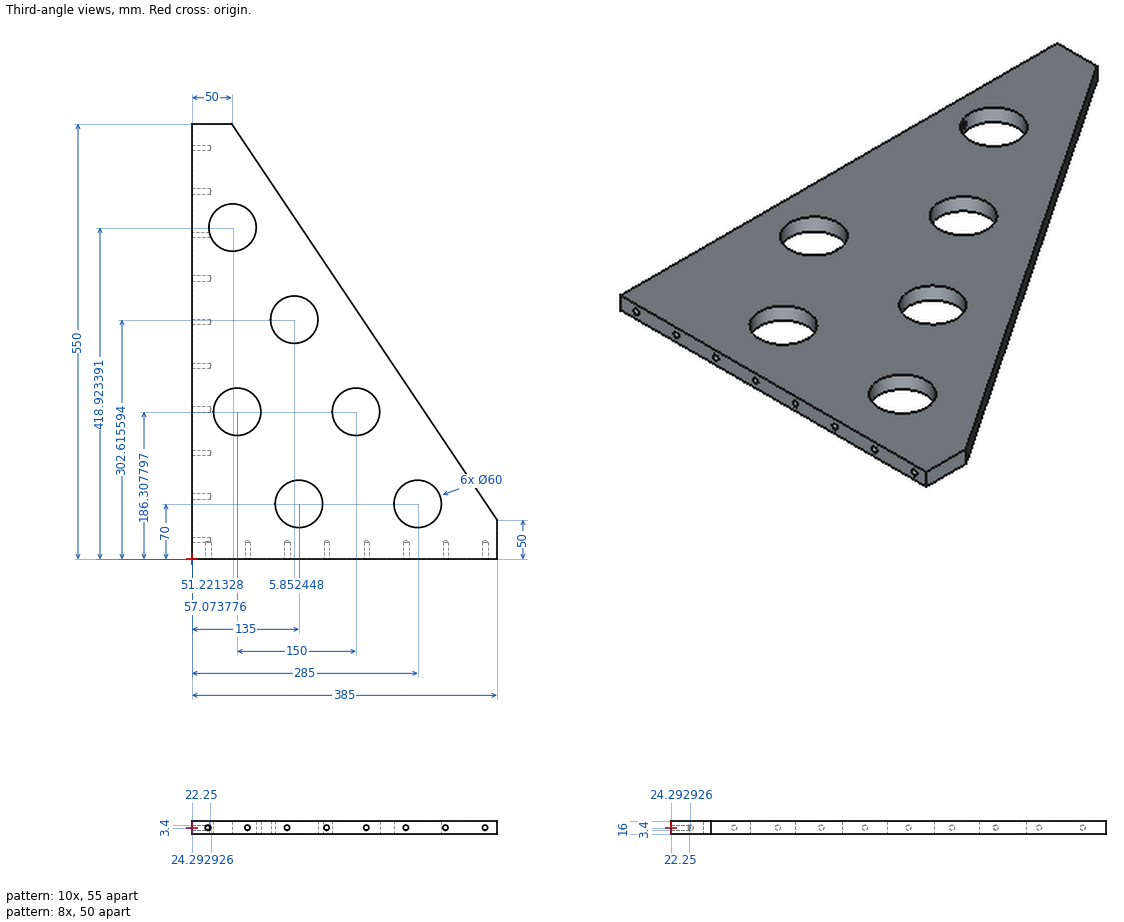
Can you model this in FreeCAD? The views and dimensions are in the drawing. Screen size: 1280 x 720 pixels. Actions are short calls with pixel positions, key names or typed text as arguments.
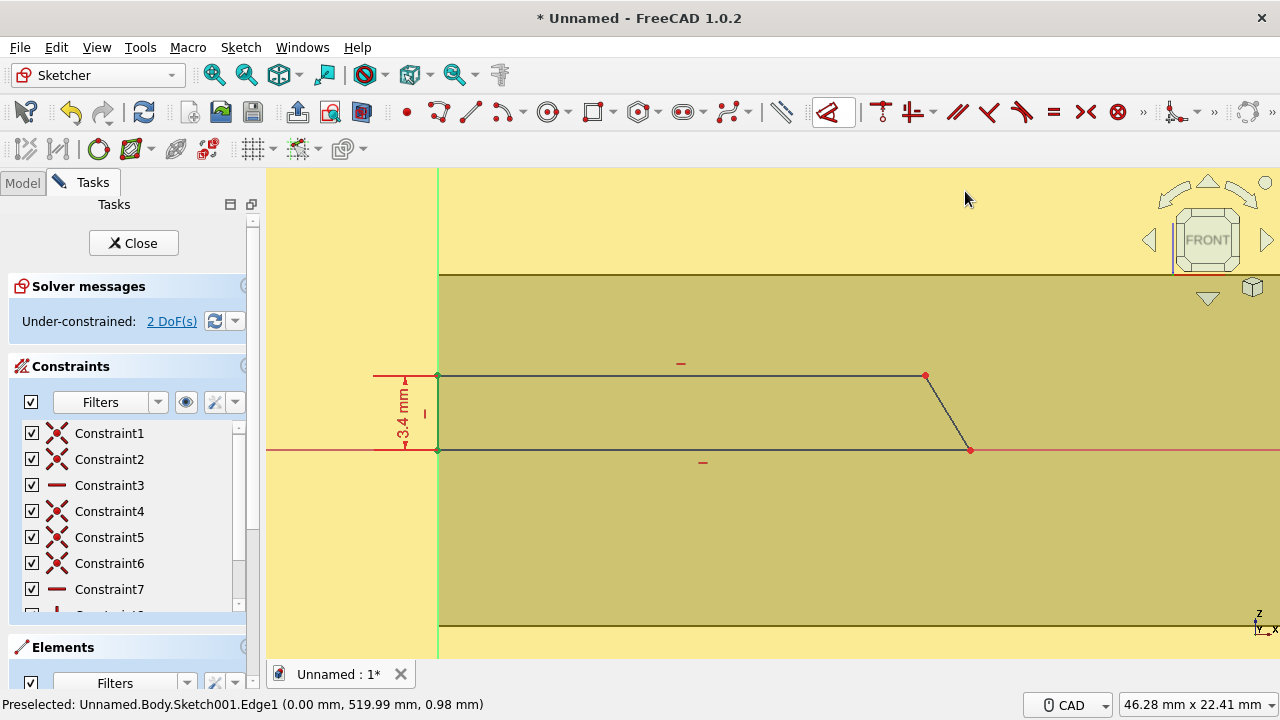
click(584, 376)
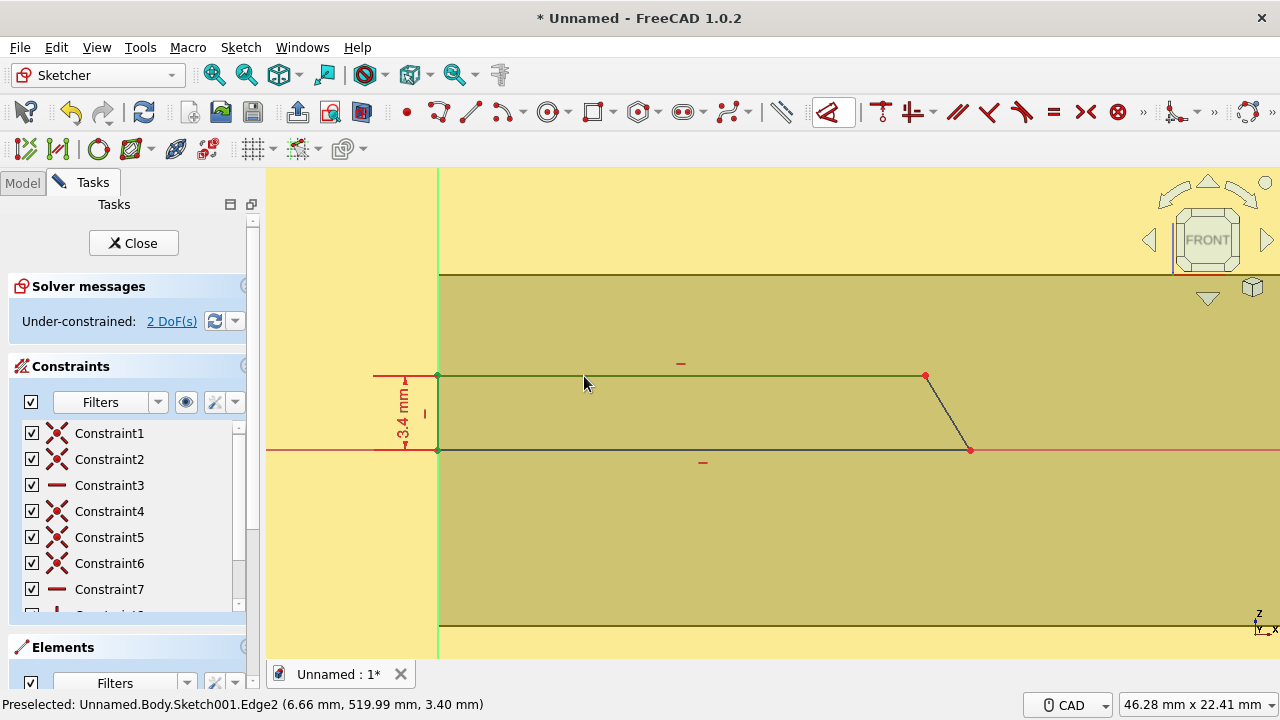
click(850, 112)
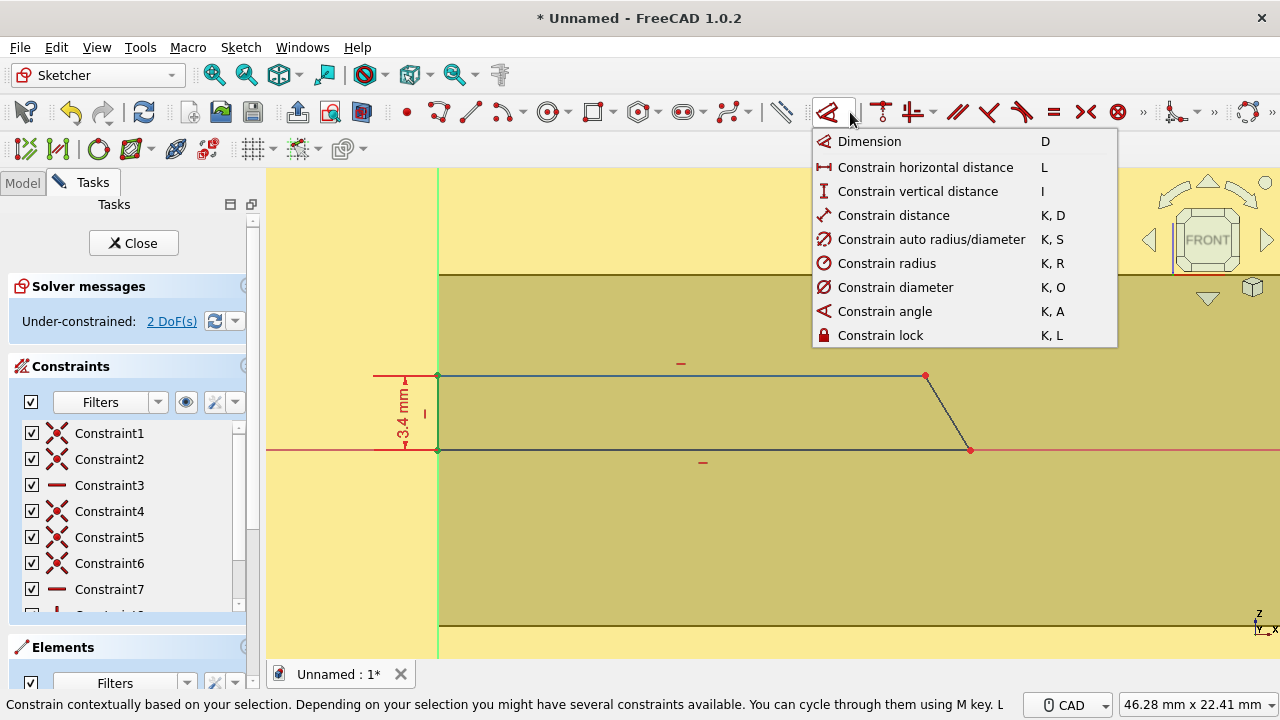
click(965, 167)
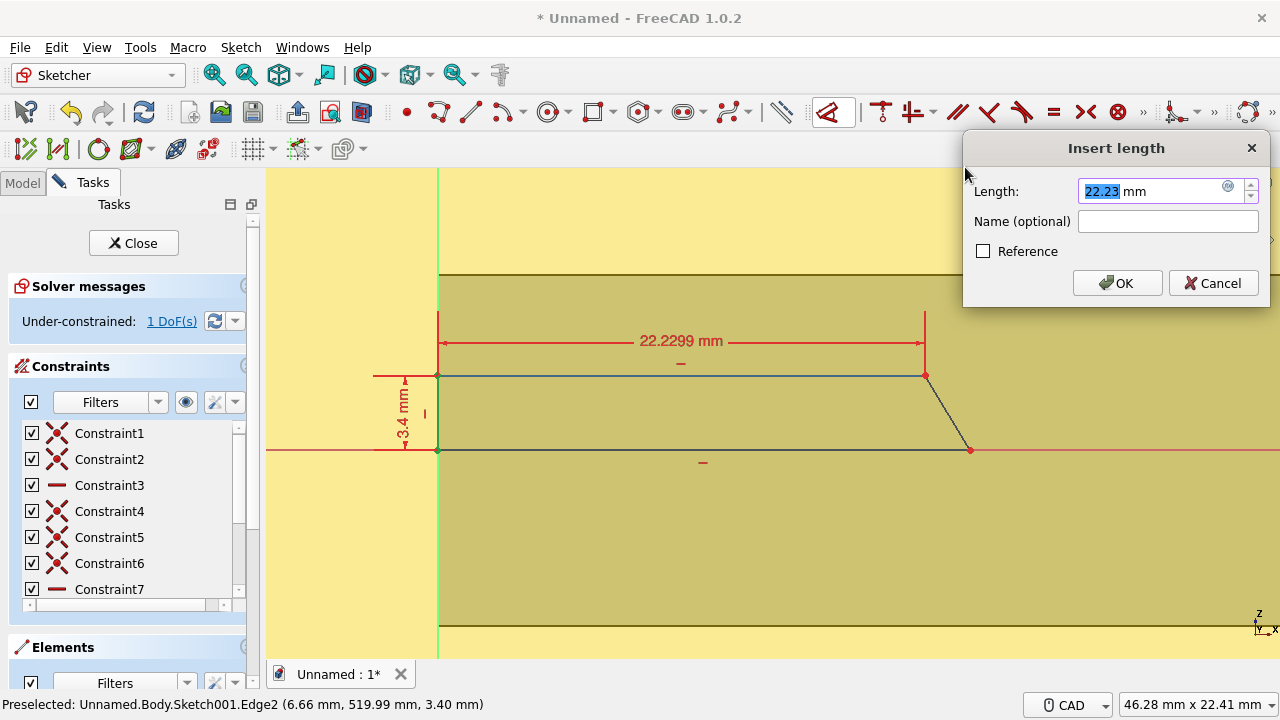
text(22.25)
key(Return)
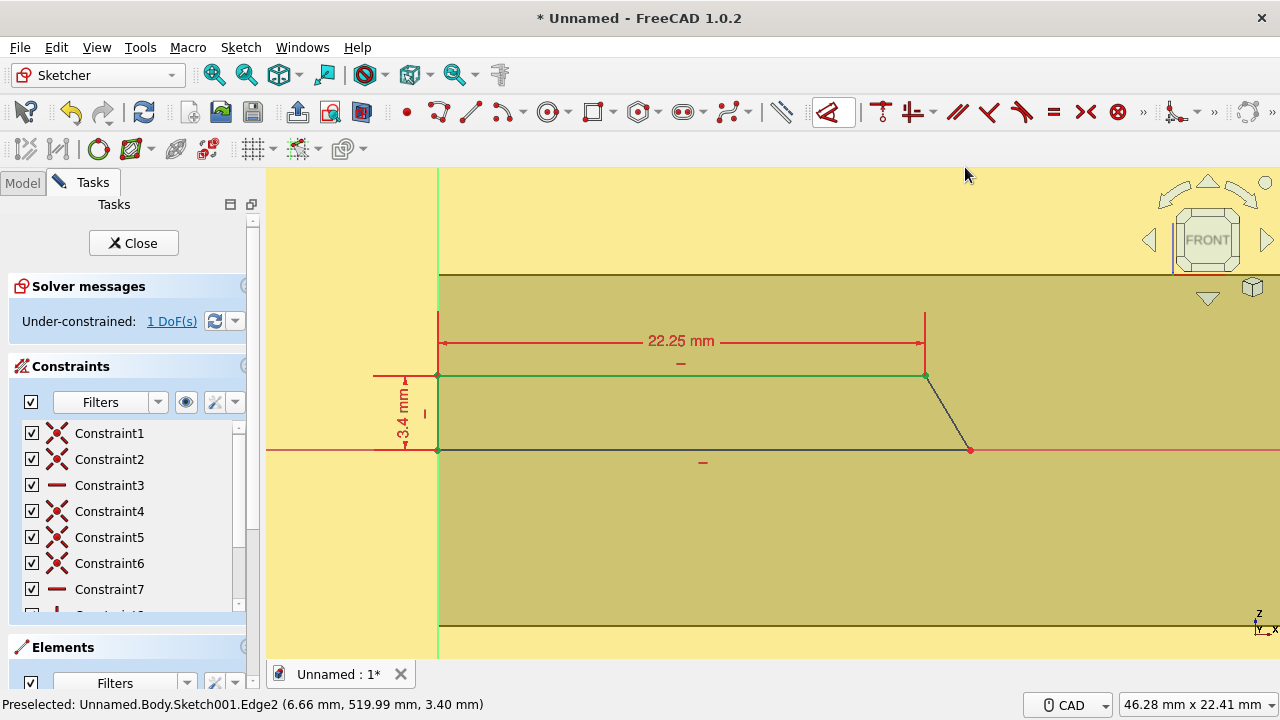
click(810, 450)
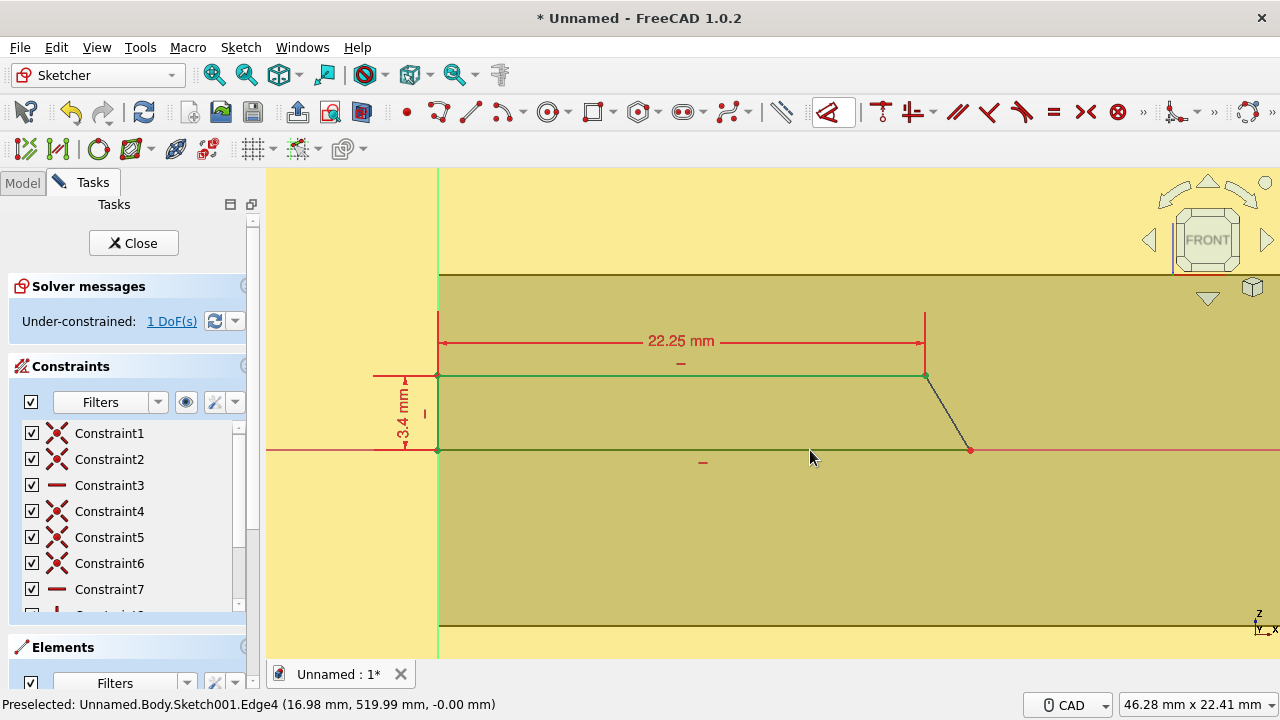
click(850, 112)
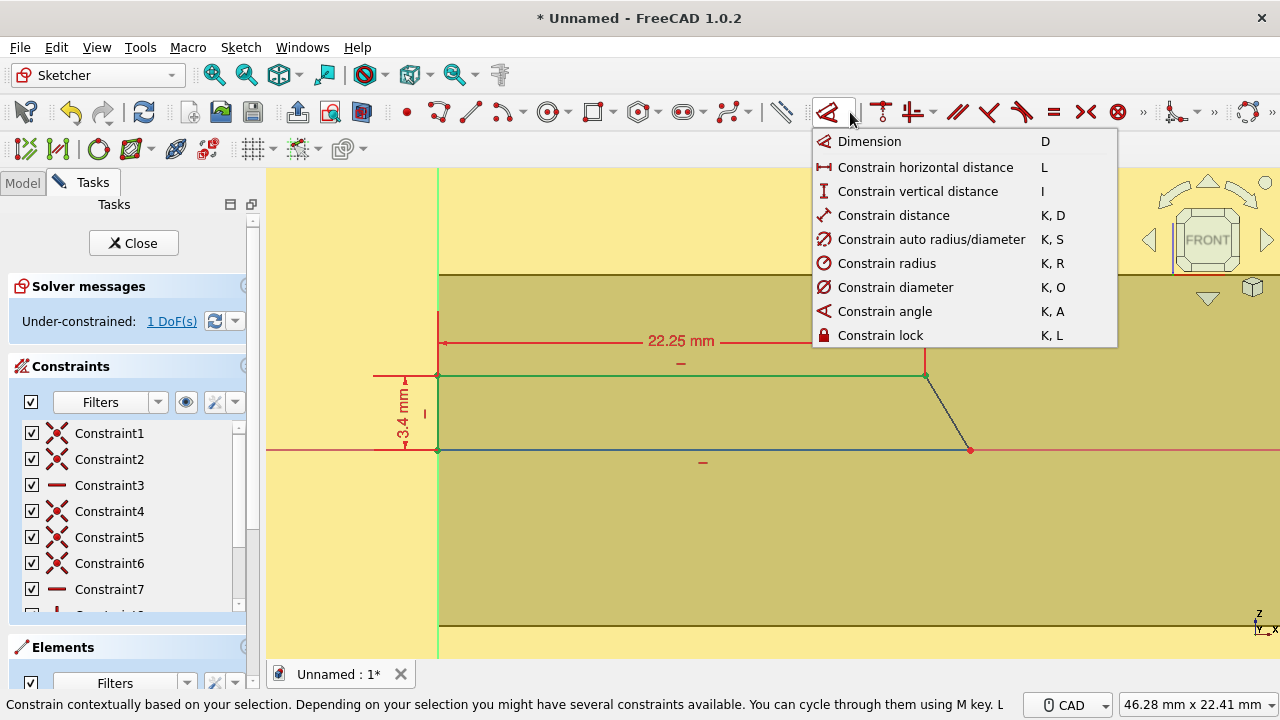
click(965, 167)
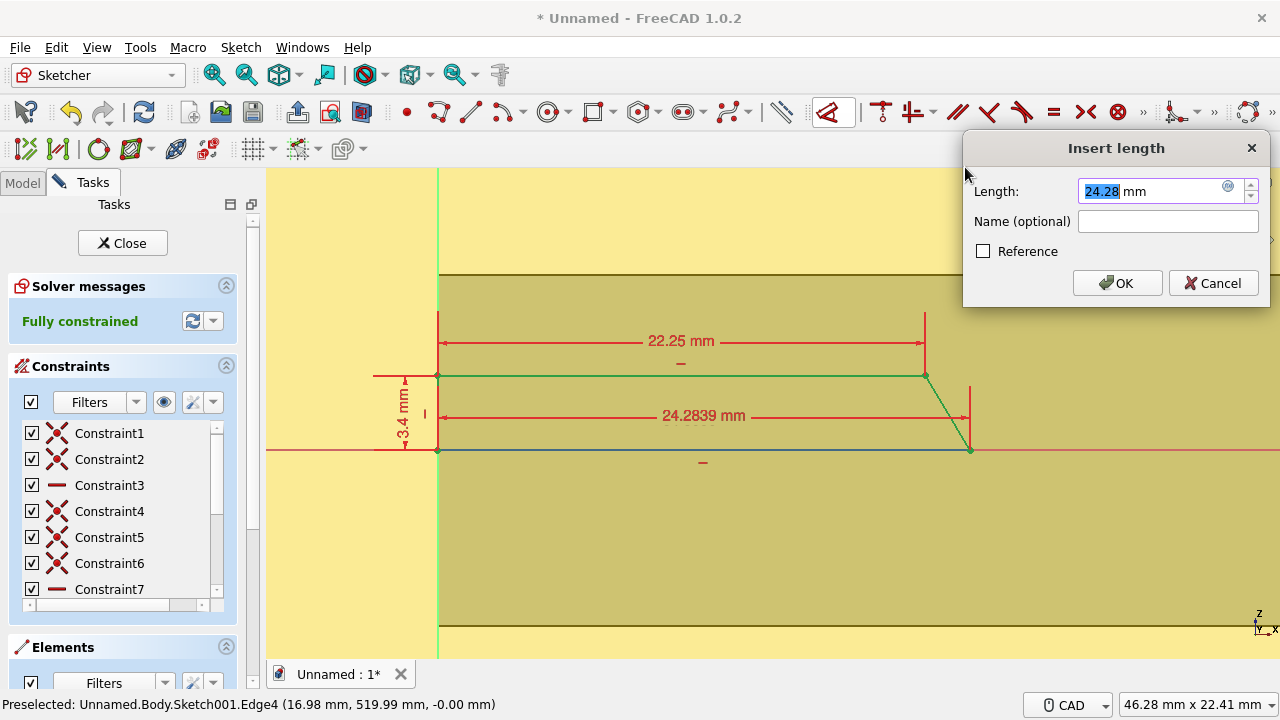
text(24.292926)
key(Return)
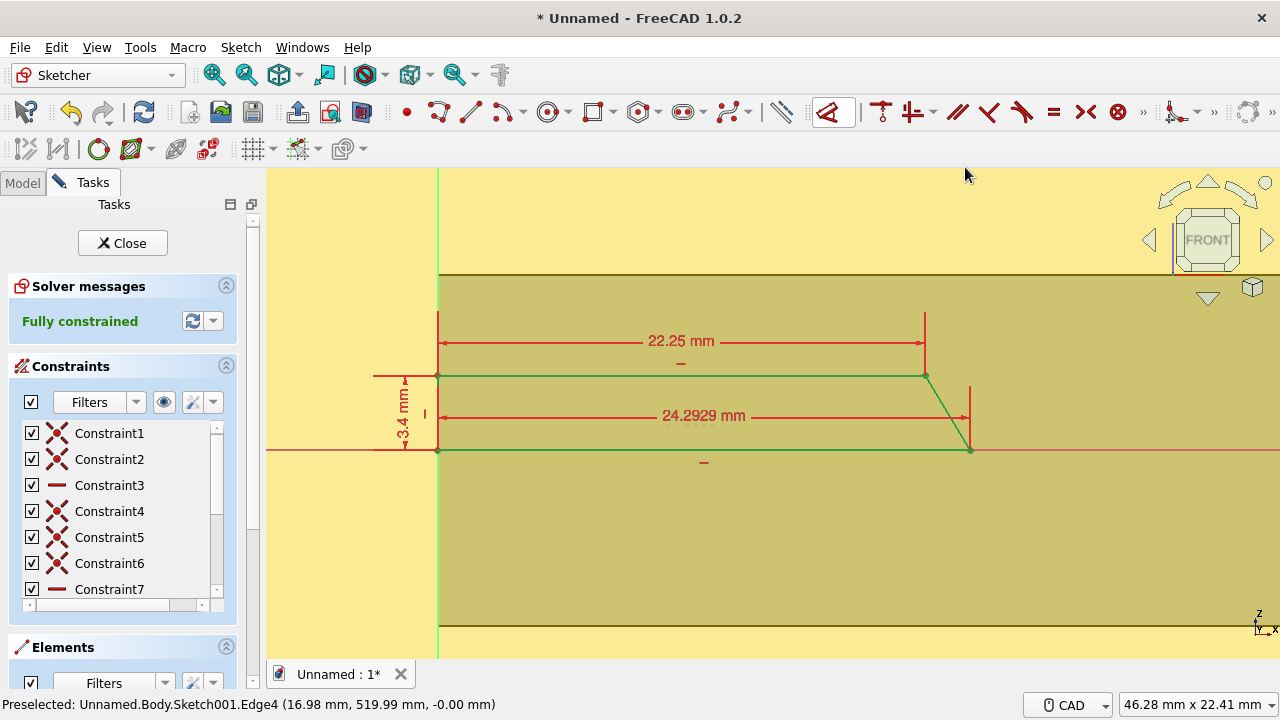
click(123, 243)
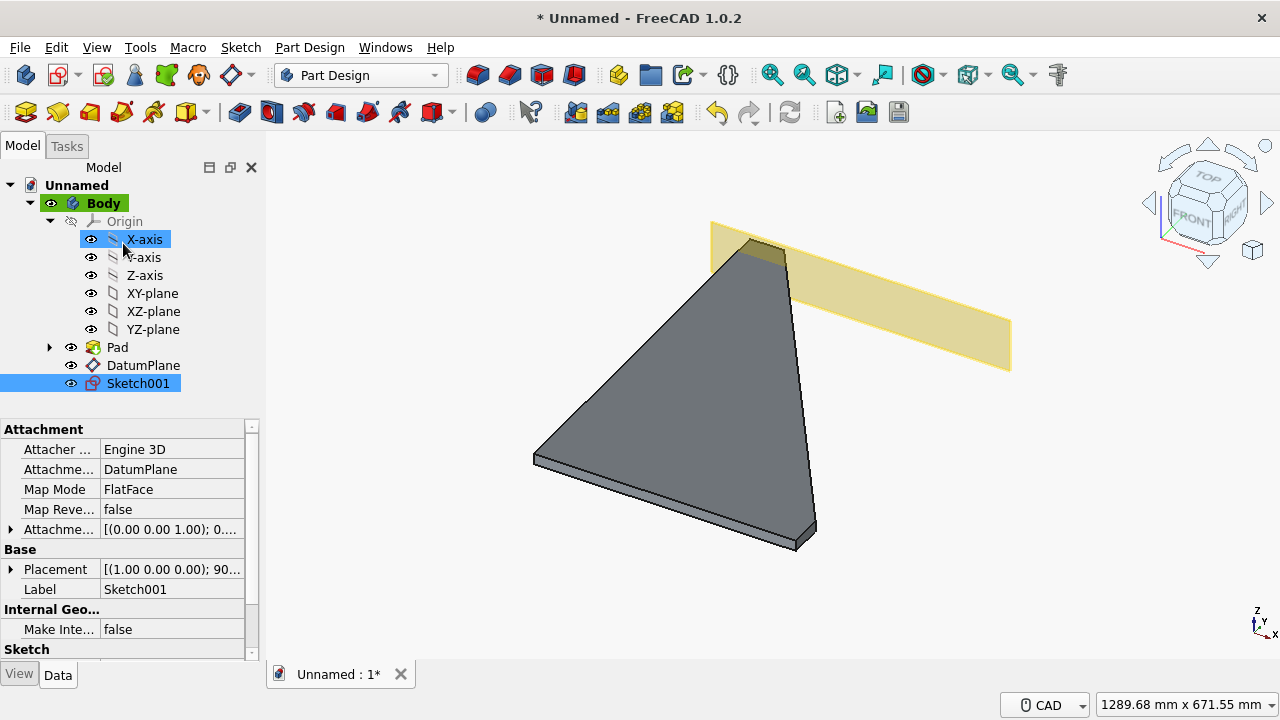
click(304, 112)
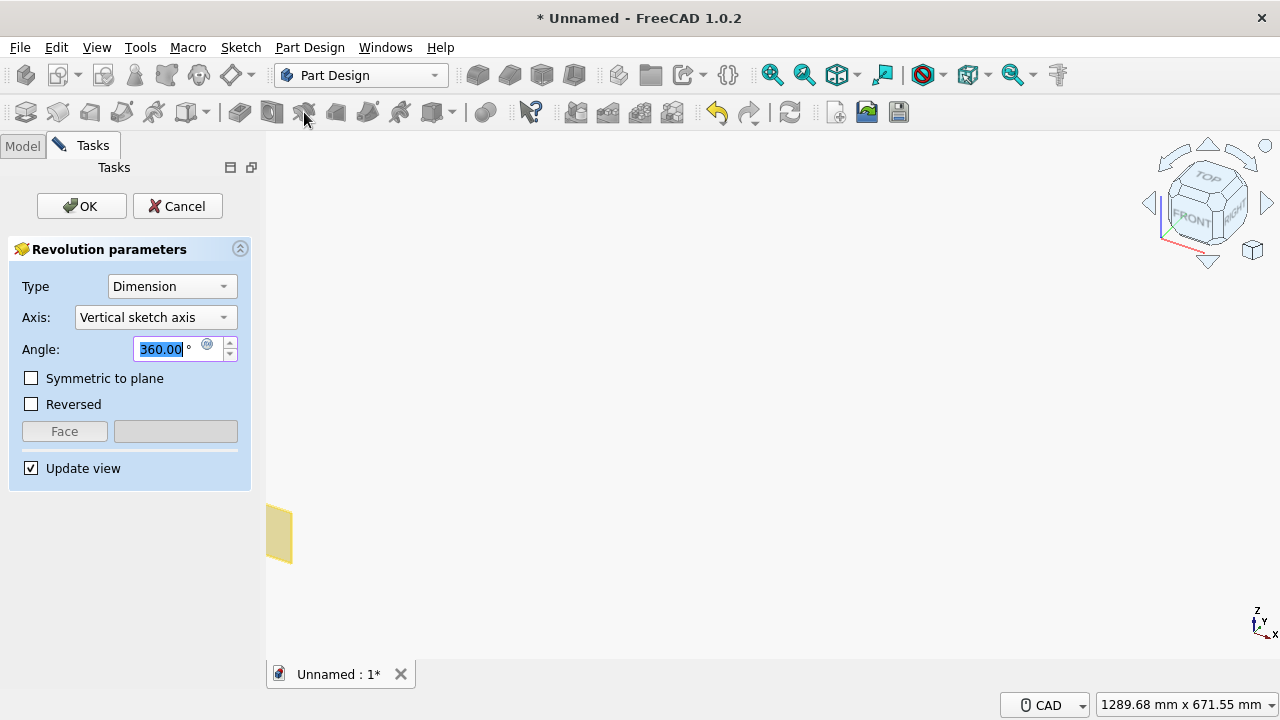
click(156, 318)